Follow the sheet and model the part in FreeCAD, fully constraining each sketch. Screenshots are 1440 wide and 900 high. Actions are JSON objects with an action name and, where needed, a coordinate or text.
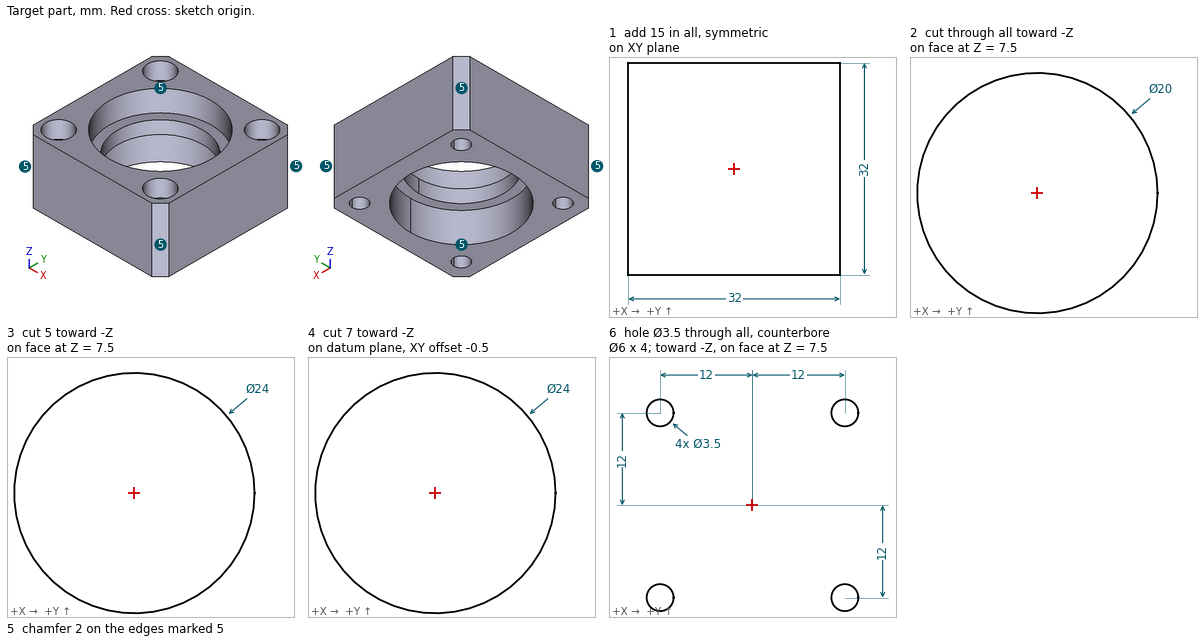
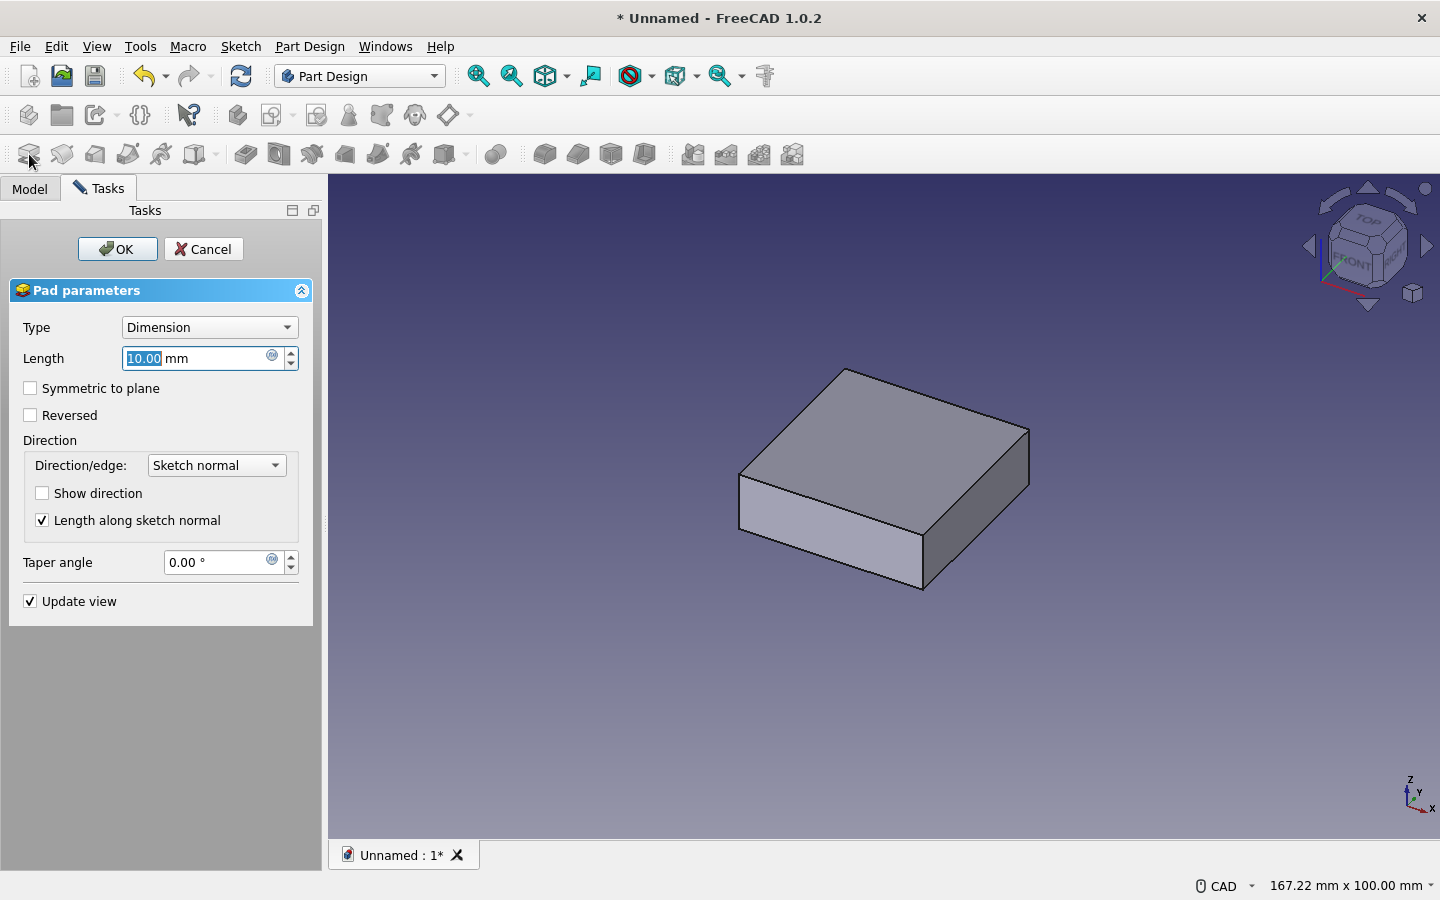
{"action": "type", "text": "15"}
{"action": "key", "text": "Tab"}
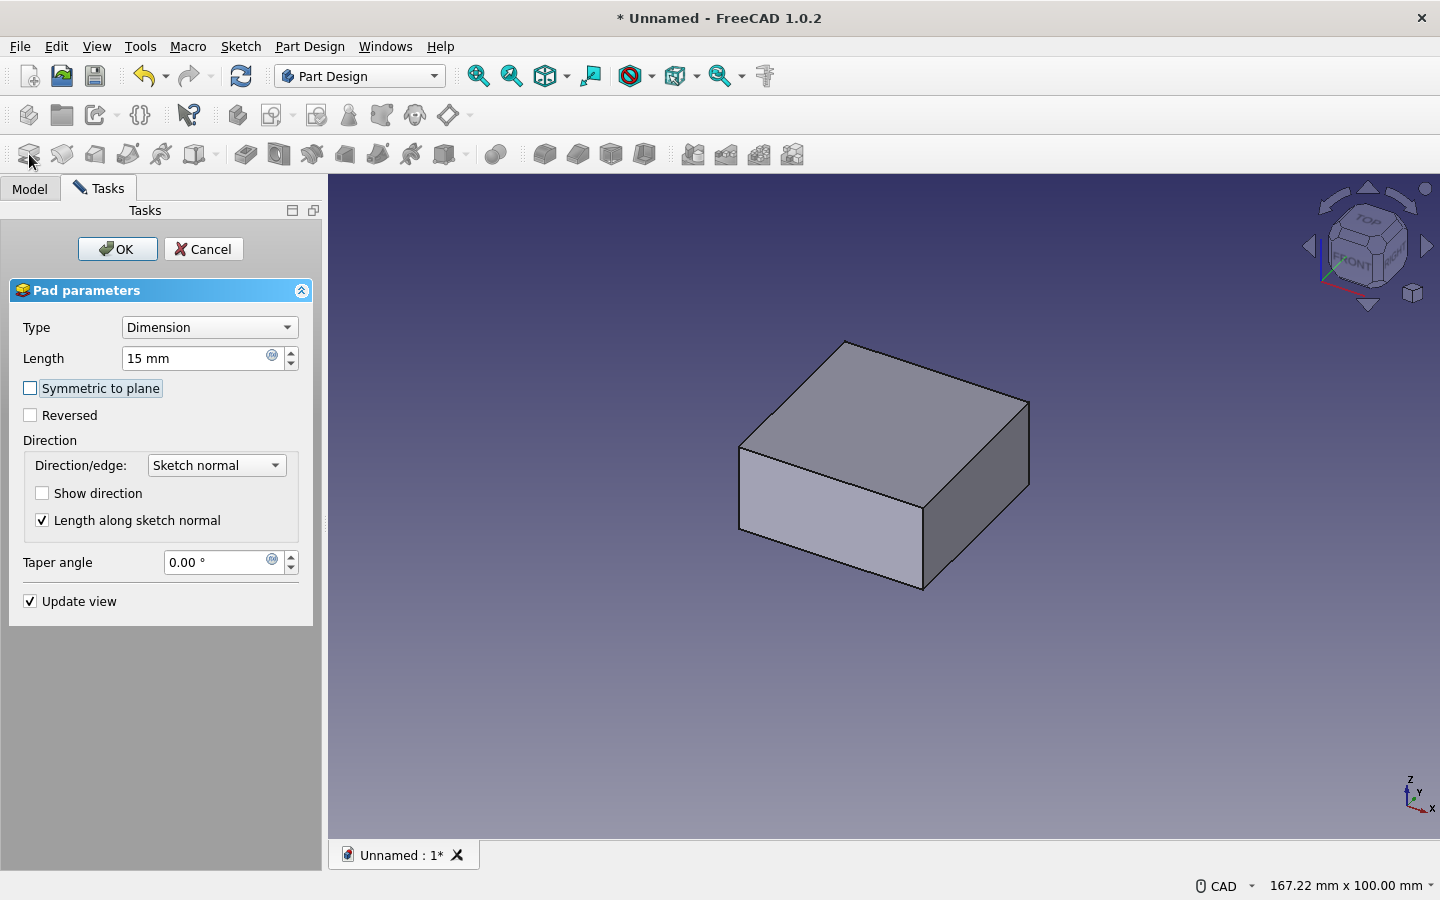
{"action": "left_click", "coordinate": [31, 388]}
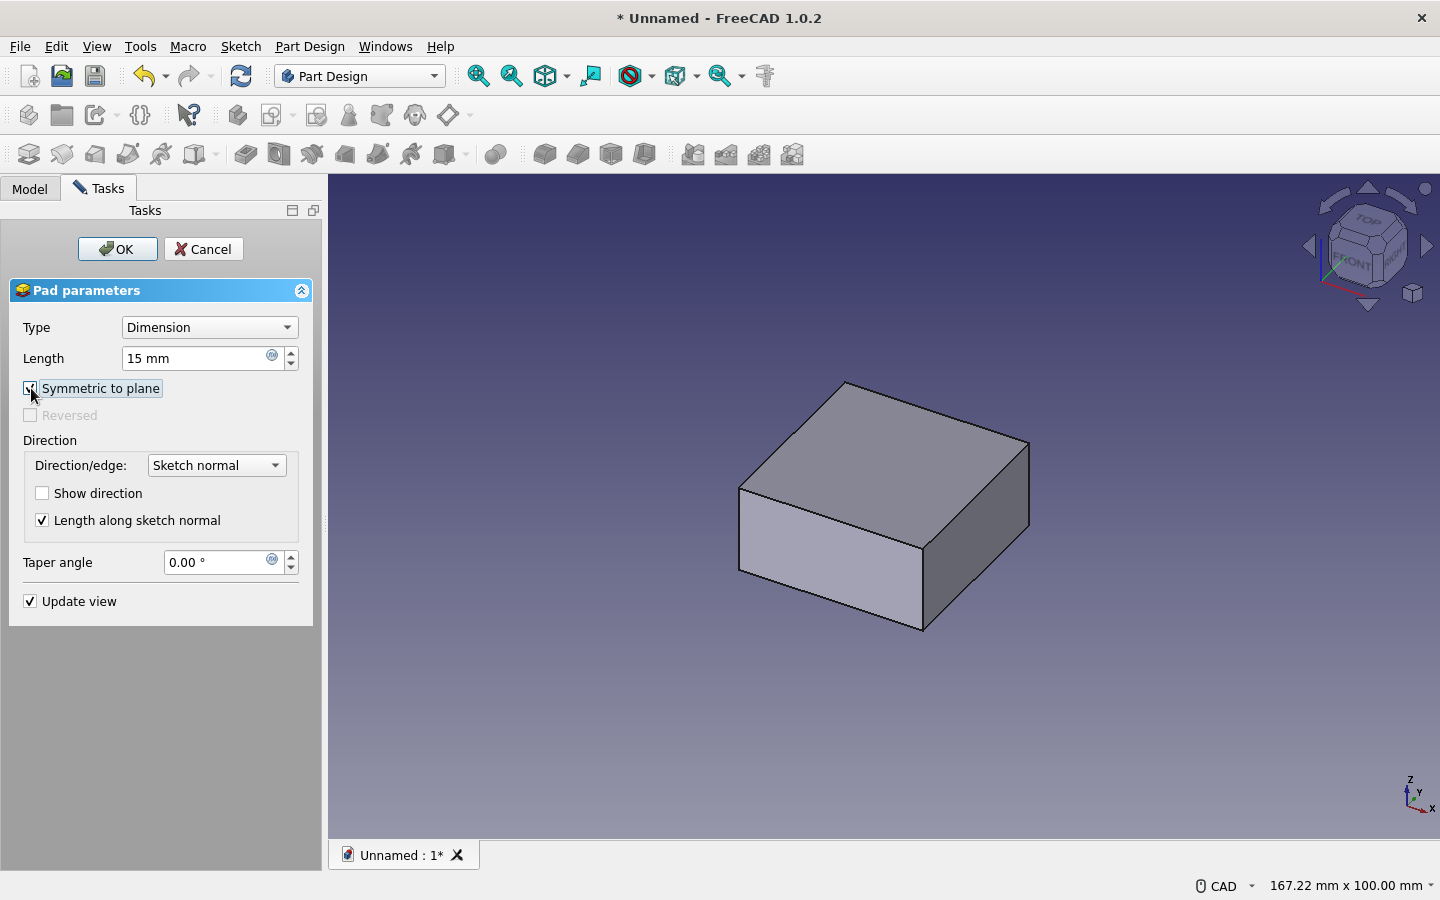
{"action": "left_click", "coordinate": [118, 249]}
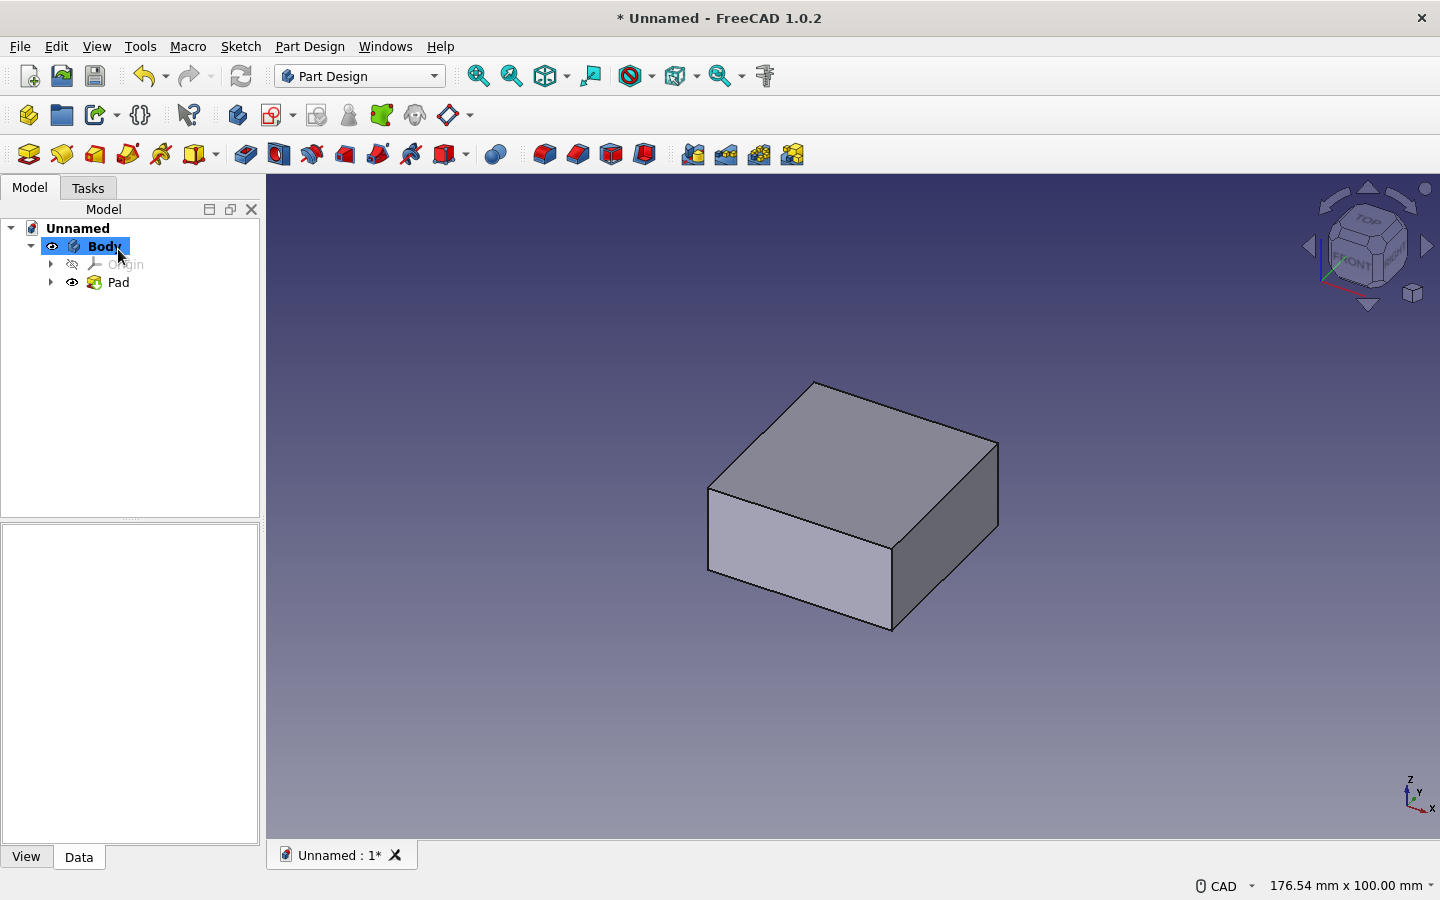
{"action": "key", "text": "v f"}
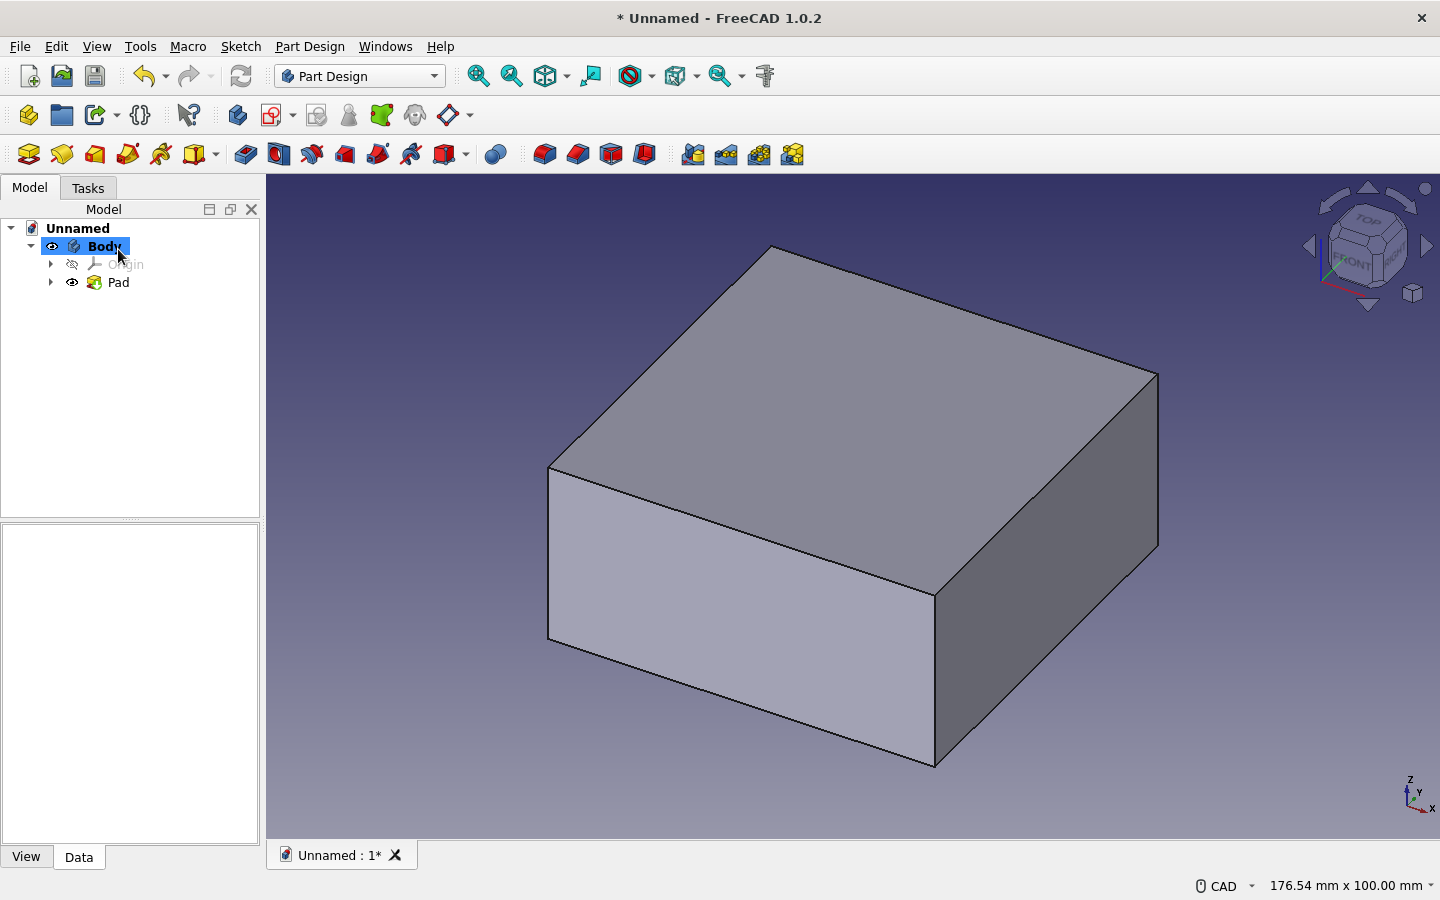
{"action": "left_click", "coordinate": [853, 420]}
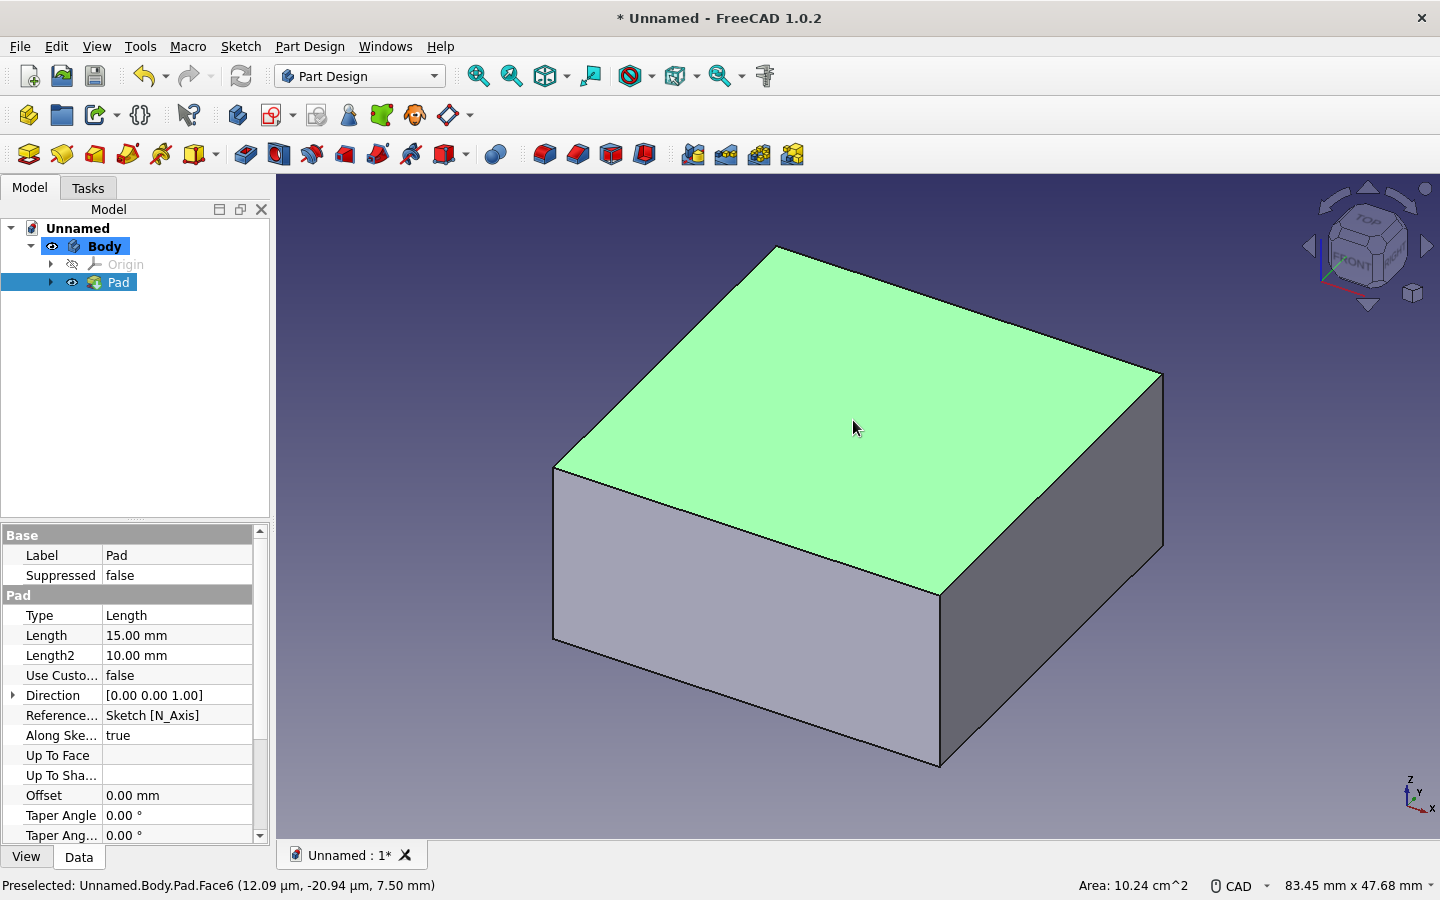
{"action": "left_click", "coordinate": [270, 116]}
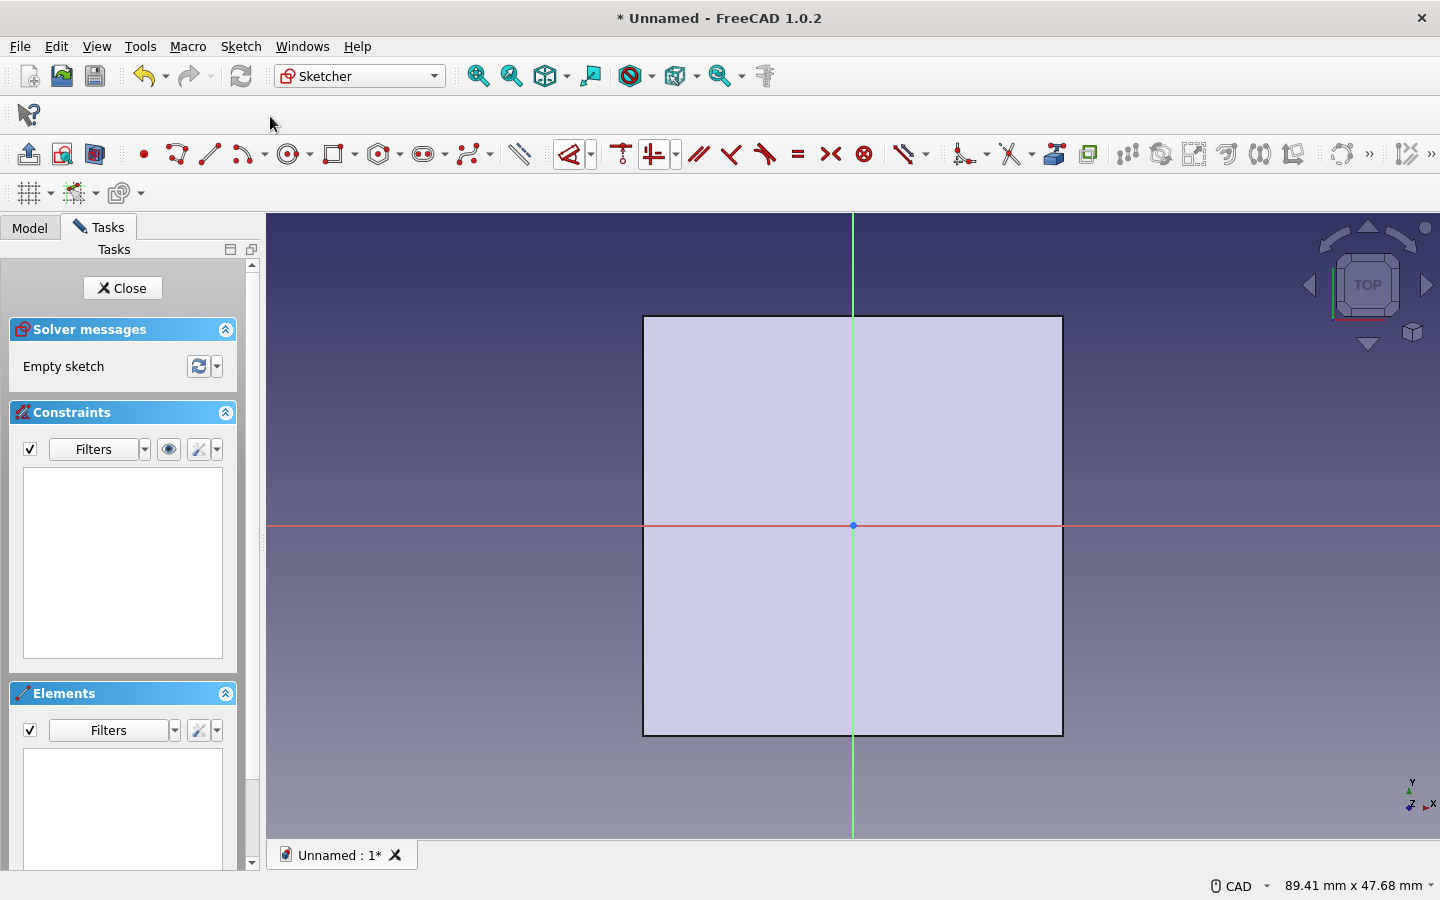
{"action": "scroll", "coordinate": [992, 526], "scroll_direction": "up", "scroll_amount": 2}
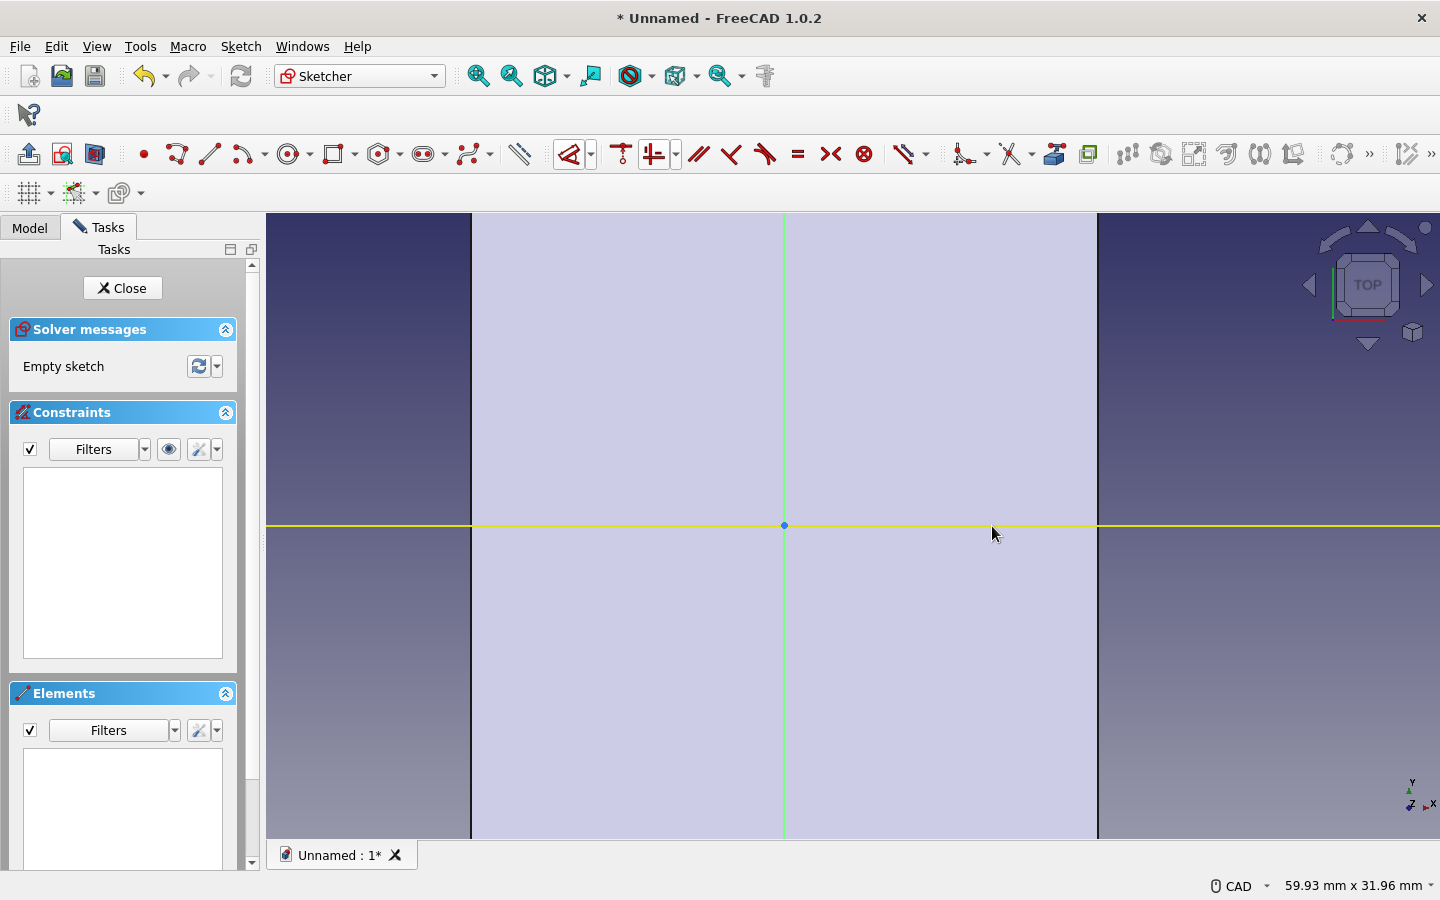
{"action": "left_click", "coordinate": [288, 154]}